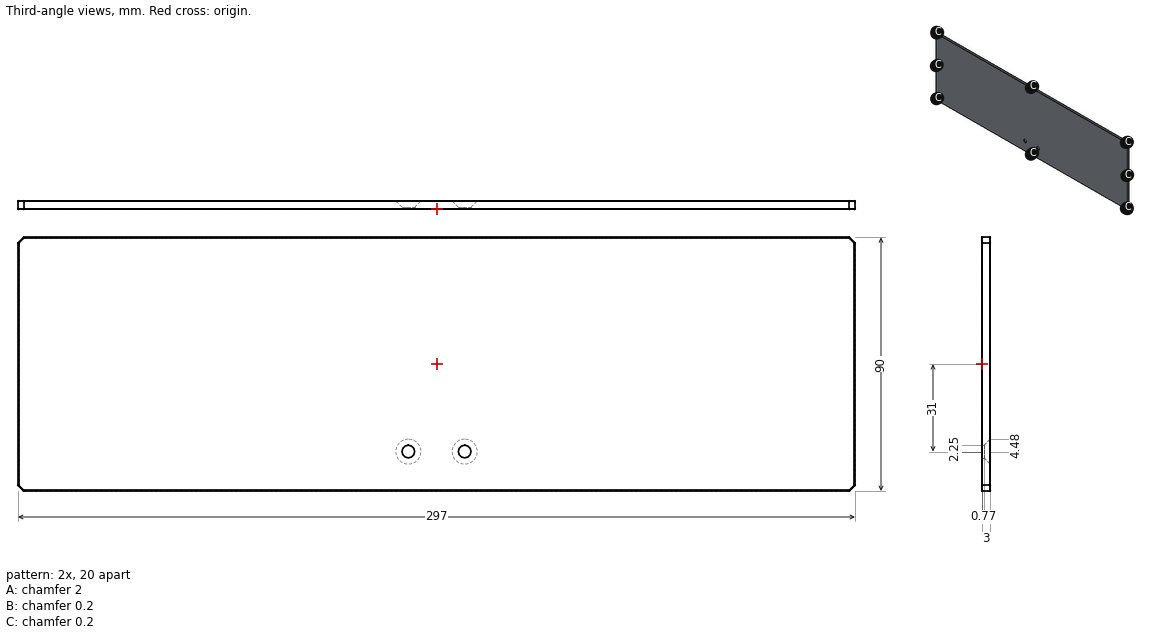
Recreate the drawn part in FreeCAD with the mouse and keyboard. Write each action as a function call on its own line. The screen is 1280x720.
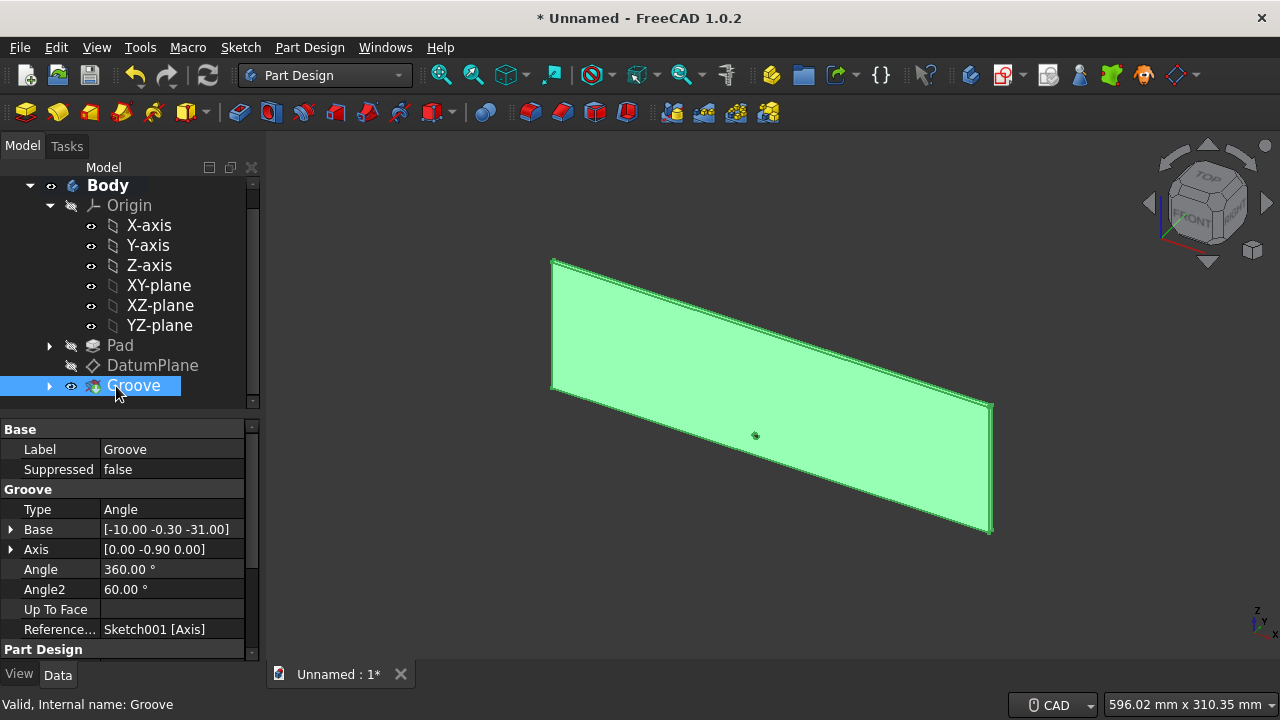
click(704, 112)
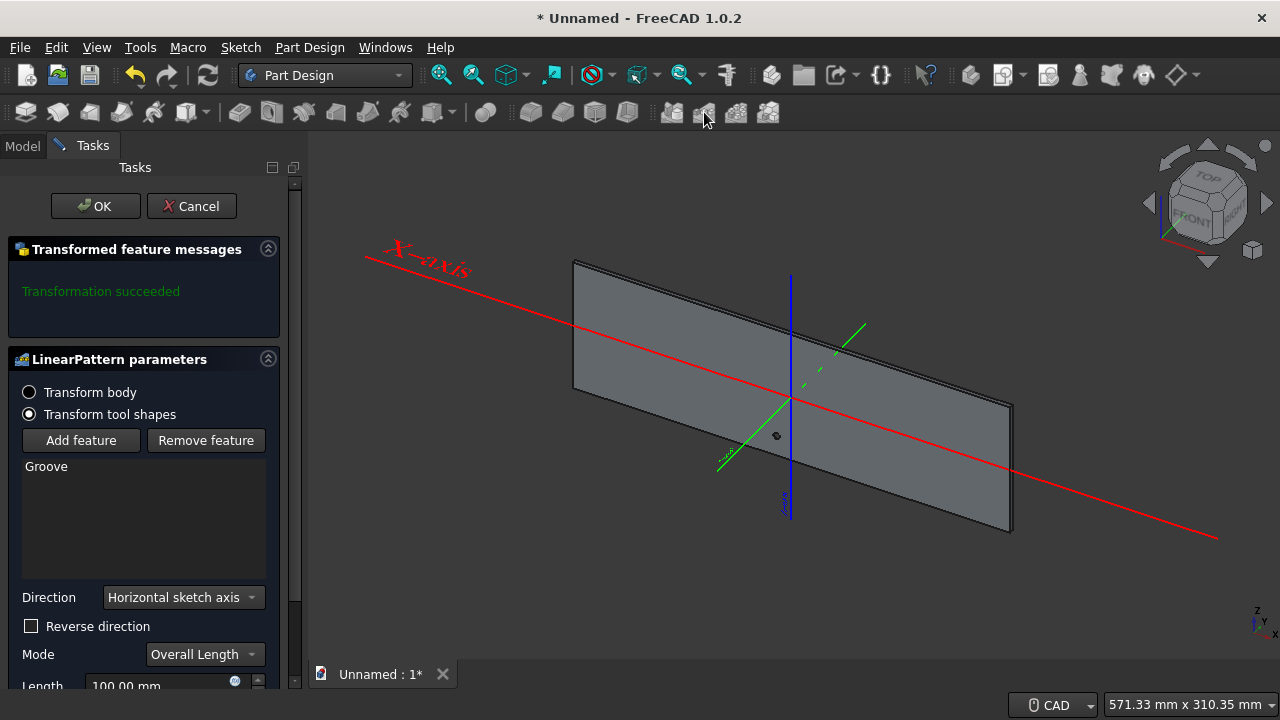
click(184, 598)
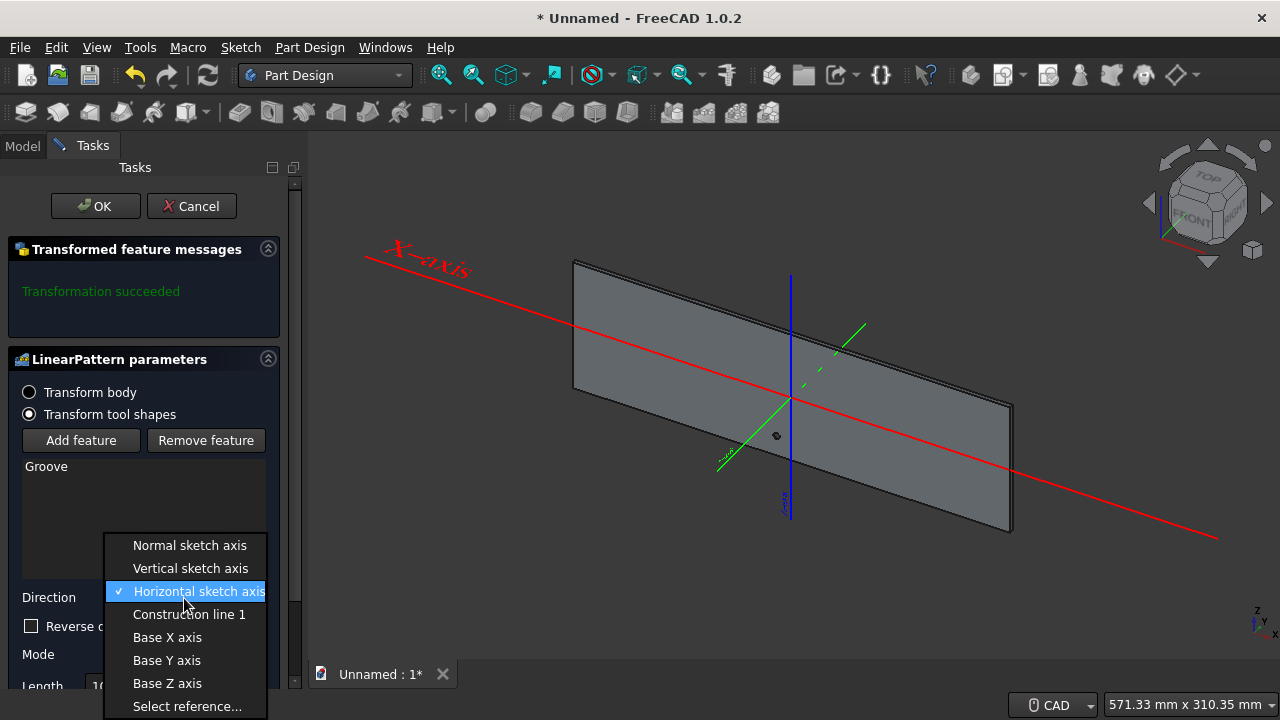
click(184, 638)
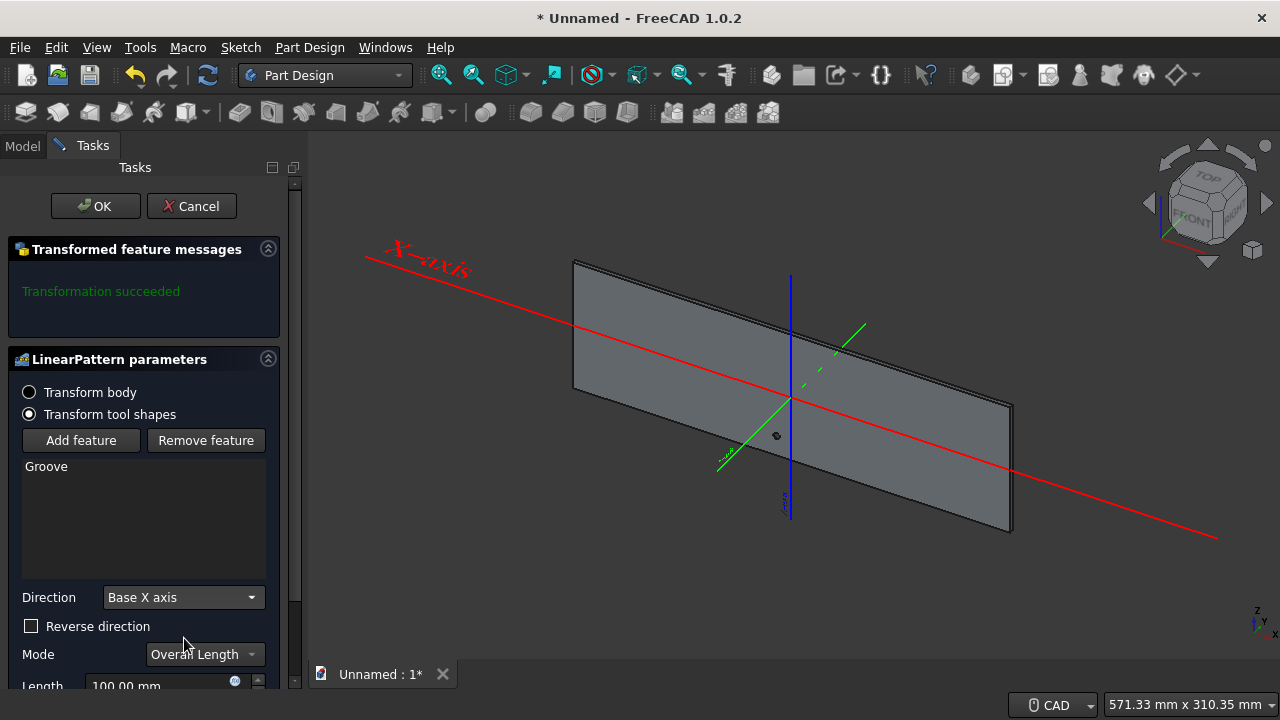
click(206, 654)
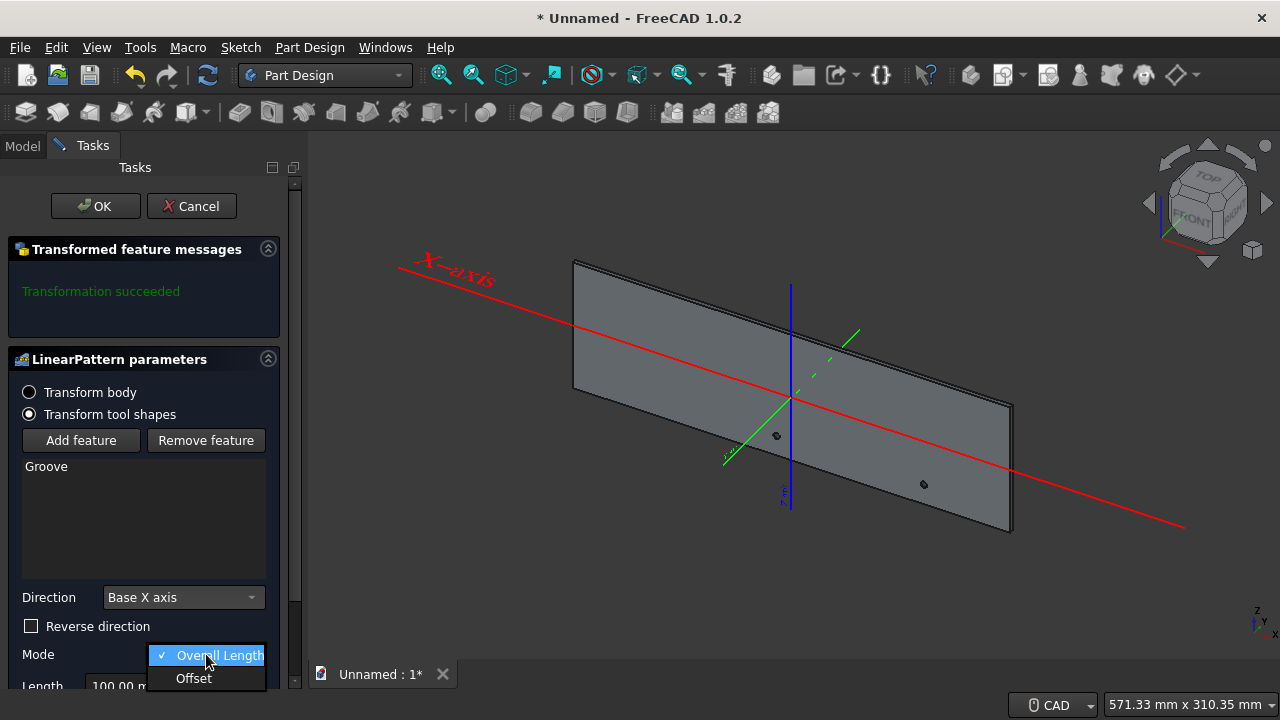
click(206, 678)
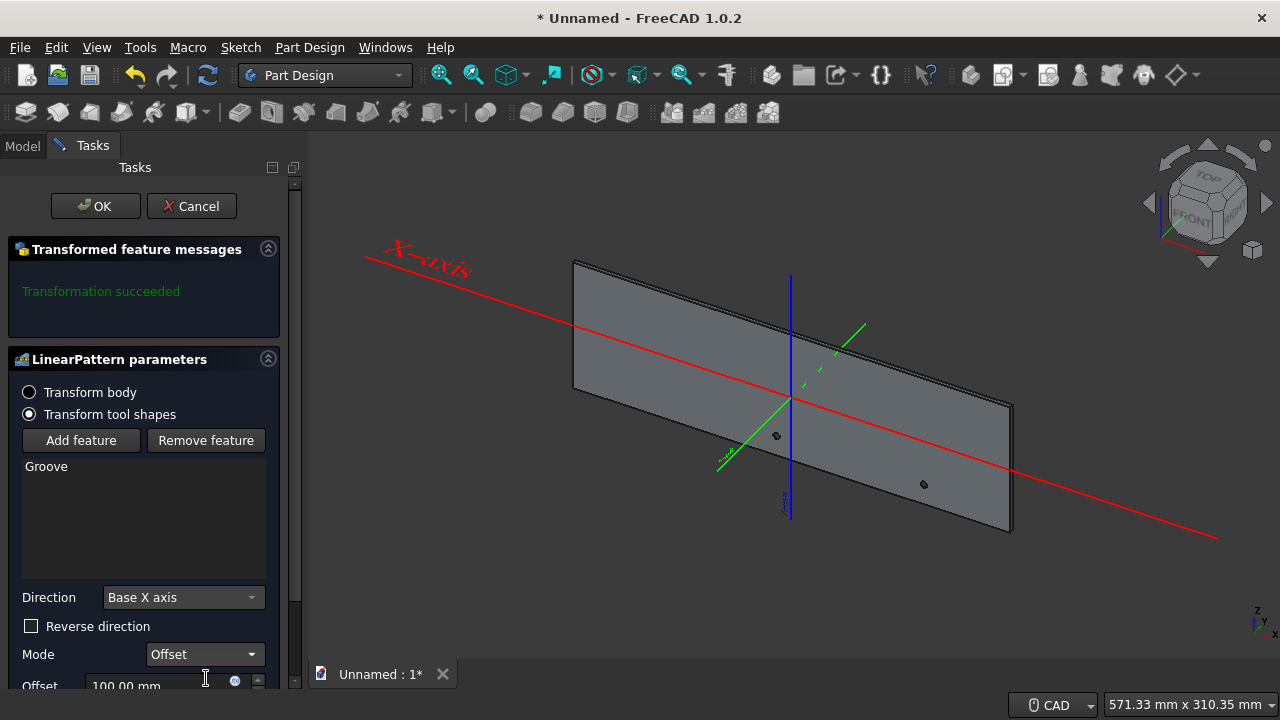
scroll(295, 432, down, 2)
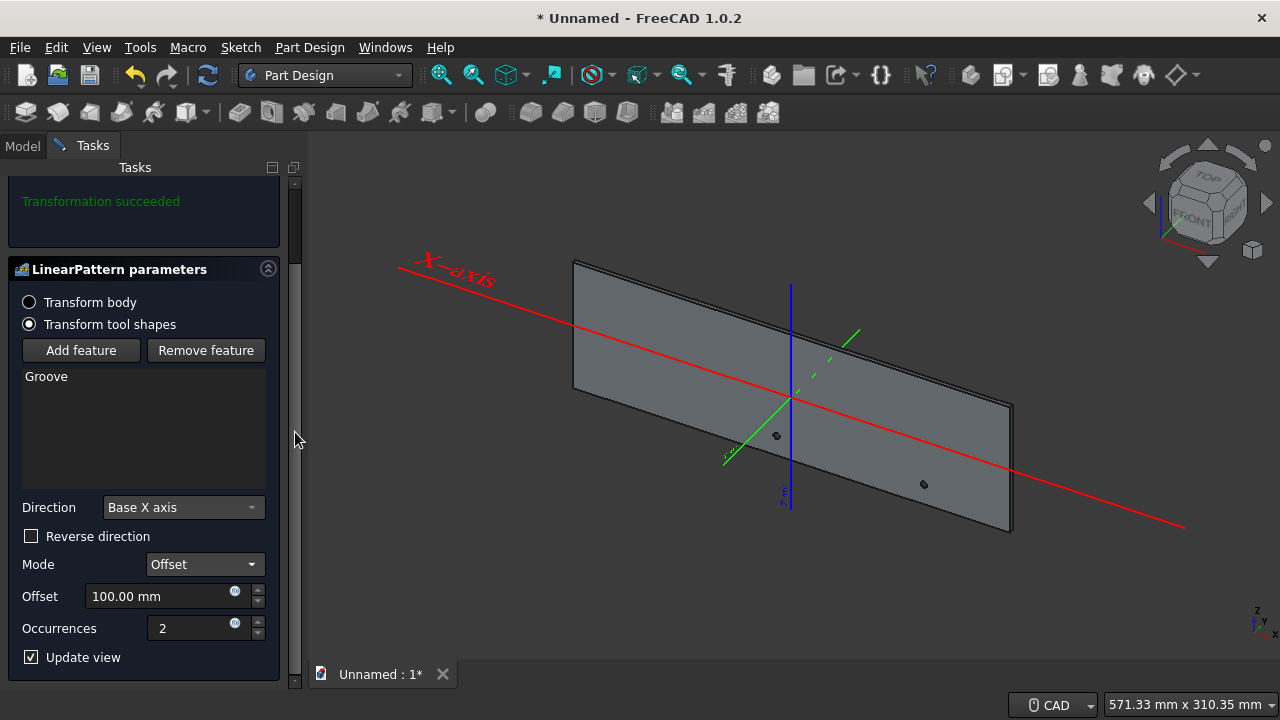
triple_click(168, 596)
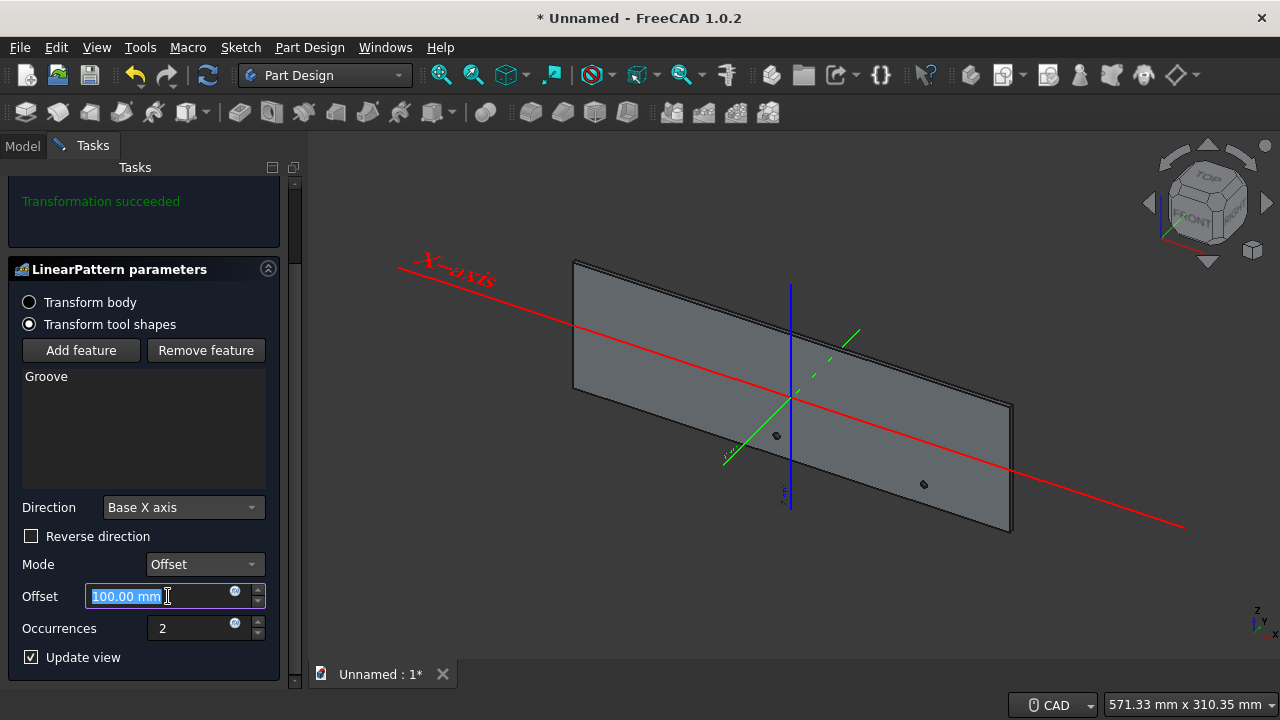
text(20)
key(Tab)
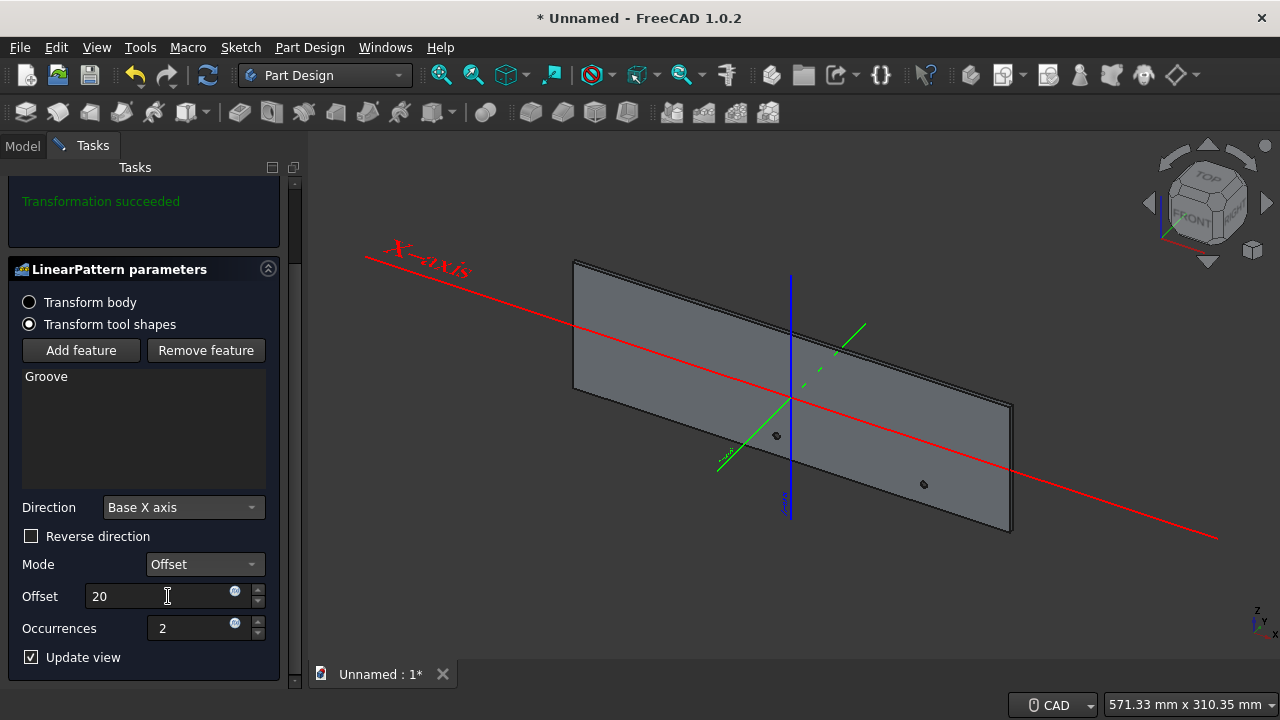
triple_click(198, 628)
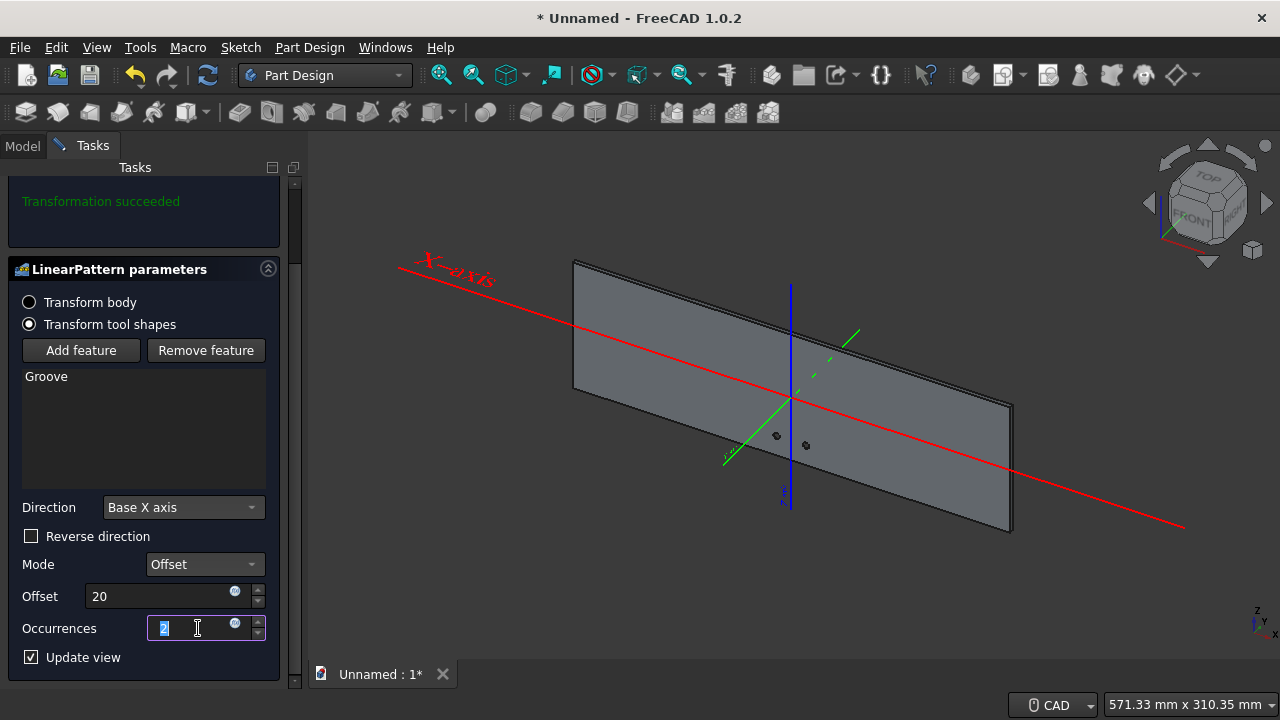
text(2)
key(Tab)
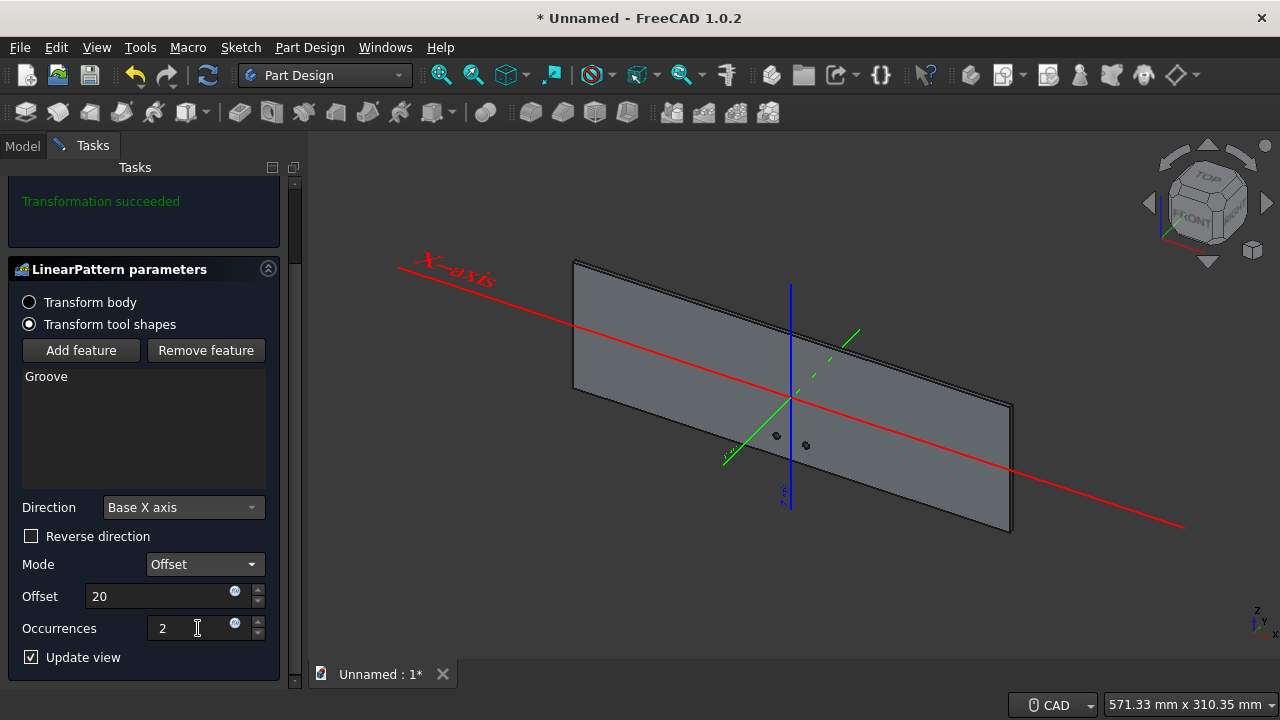
scroll(295, 432, up, 3)